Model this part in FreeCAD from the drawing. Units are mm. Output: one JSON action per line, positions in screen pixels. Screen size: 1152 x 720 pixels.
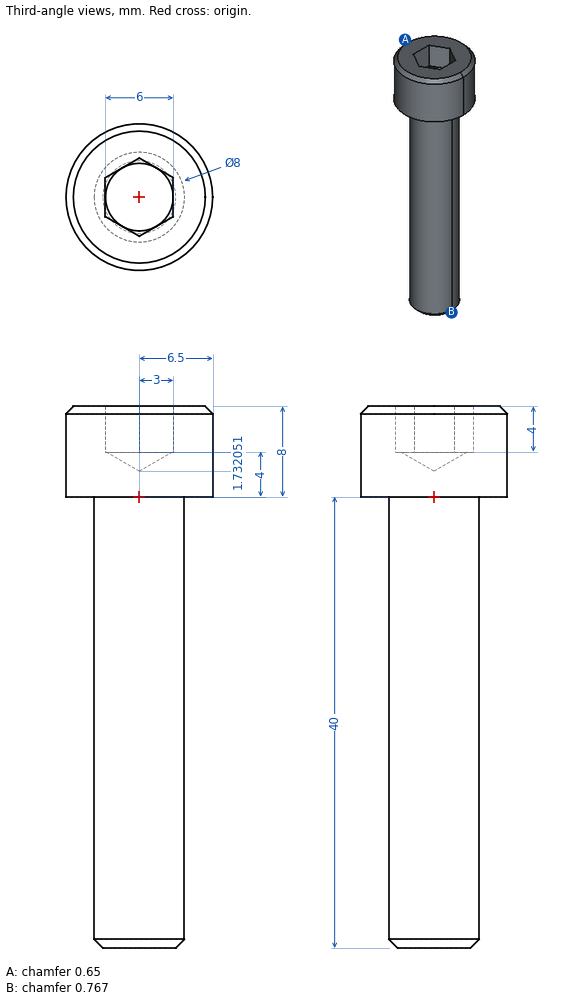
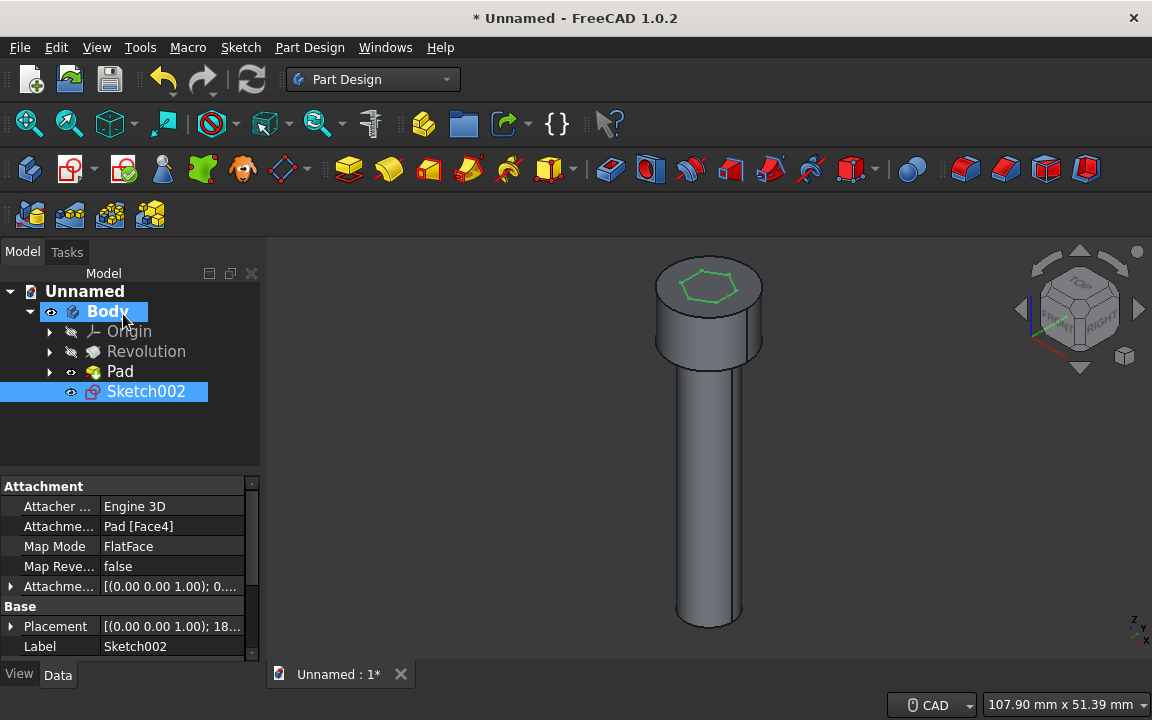
{"action": "left_click", "coordinate": [612, 170]}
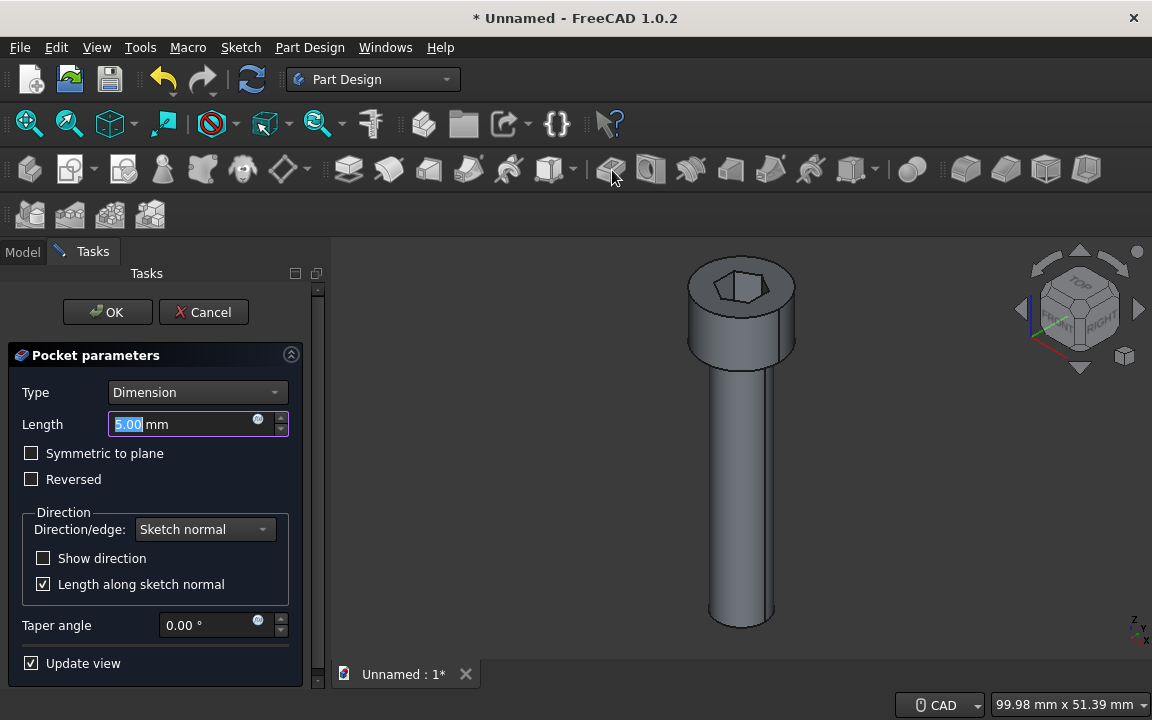
{"action": "type", "text": "4"}
{"action": "key", "text": "Tab"}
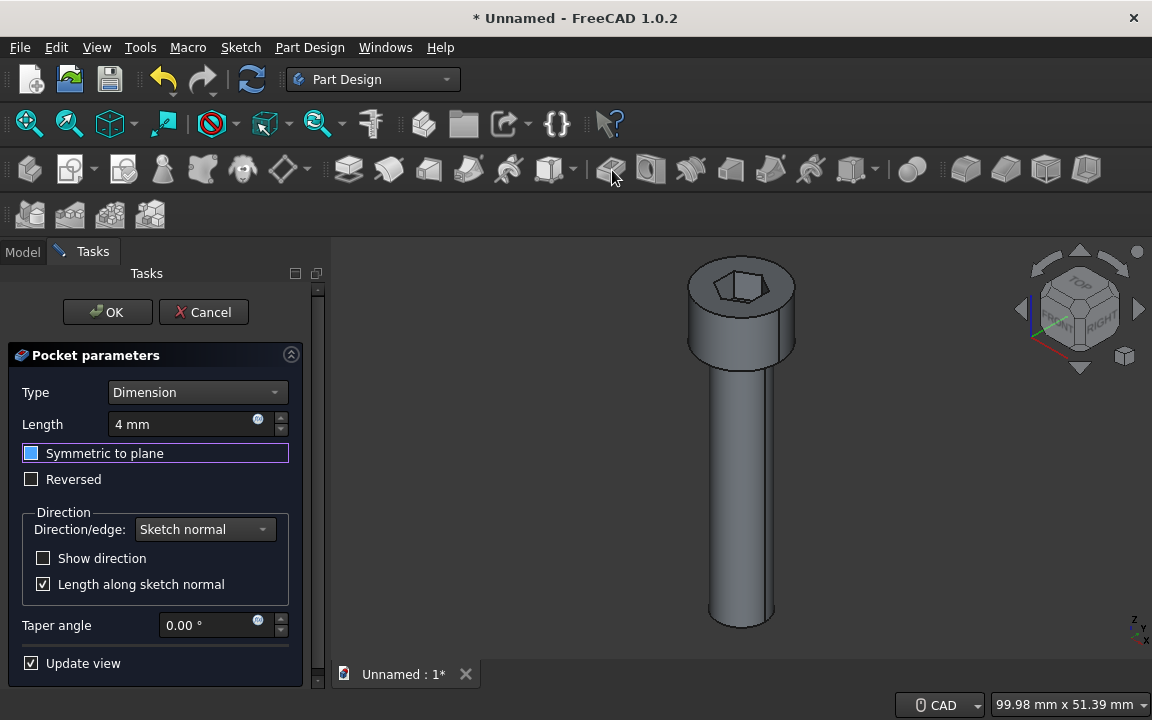
{"action": "left_click", "coordinate": [108, 312]}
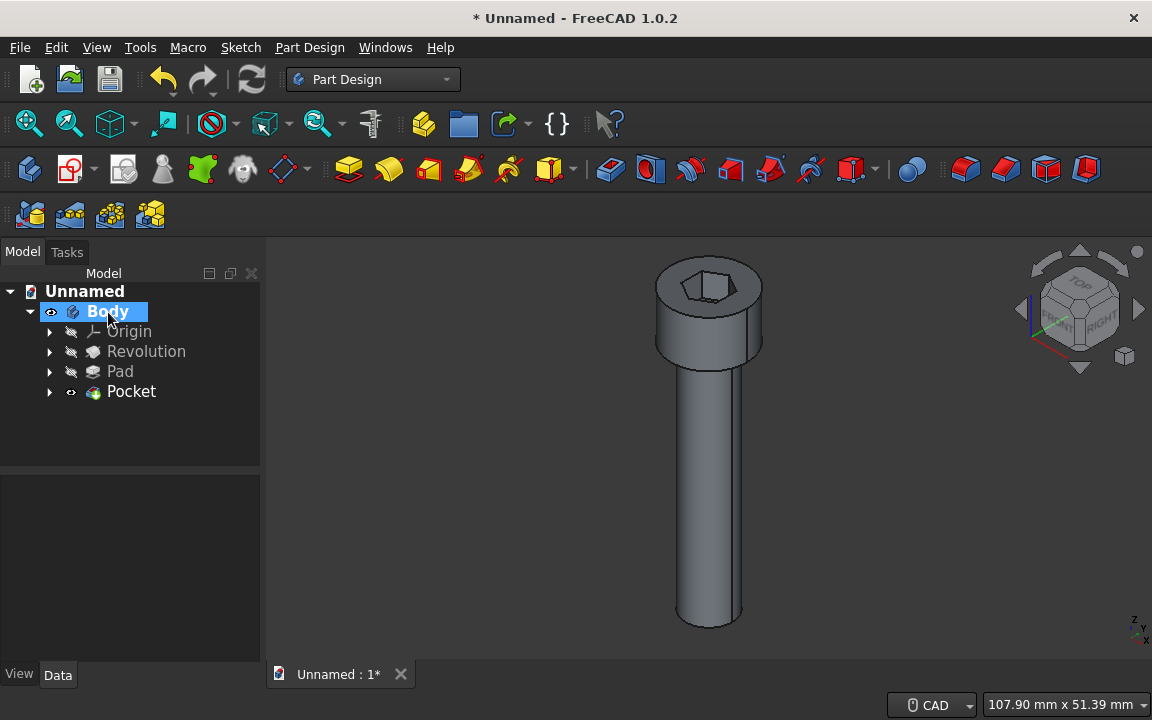
{"action": "left_click", "coordinate": [70, 170]}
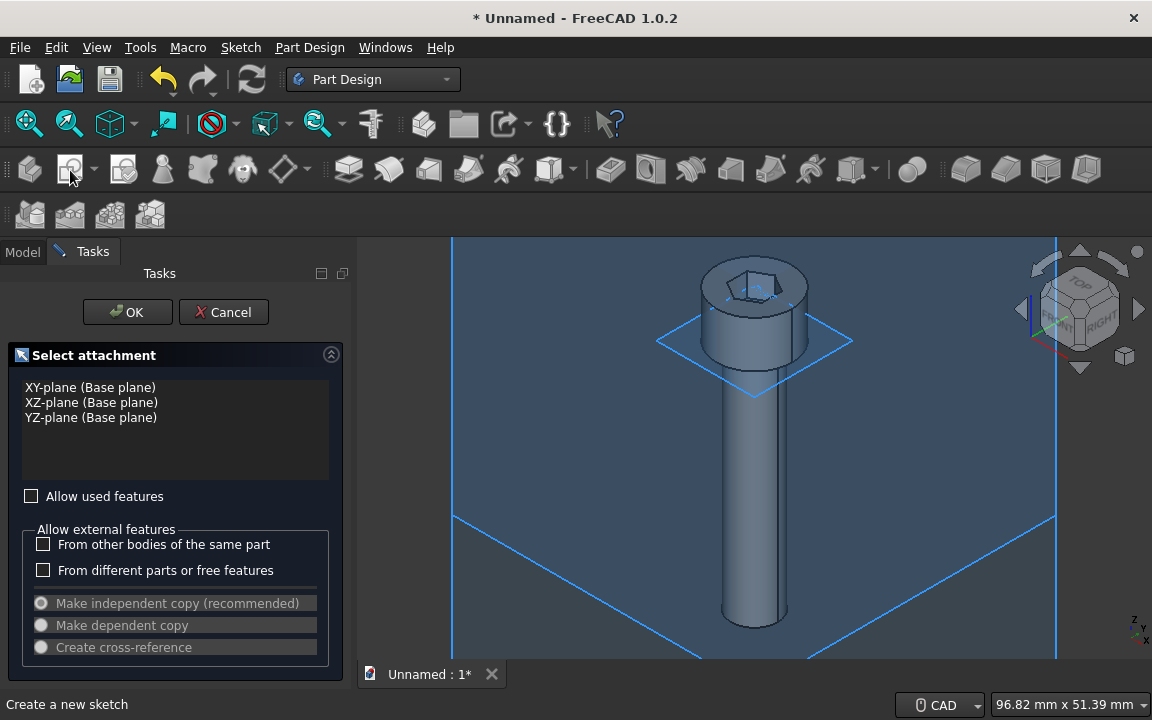
{"action": "left_click", "coordinate": [82, 402]}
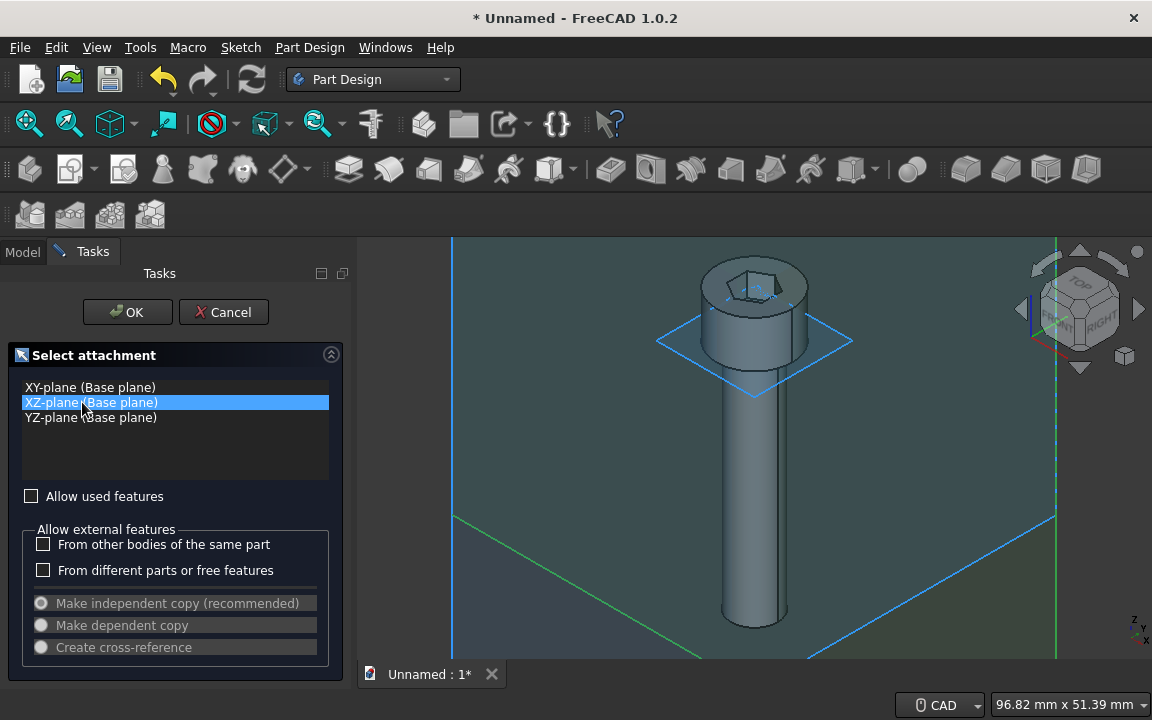
{"action": "left_click", "coordinate": [128, 312]}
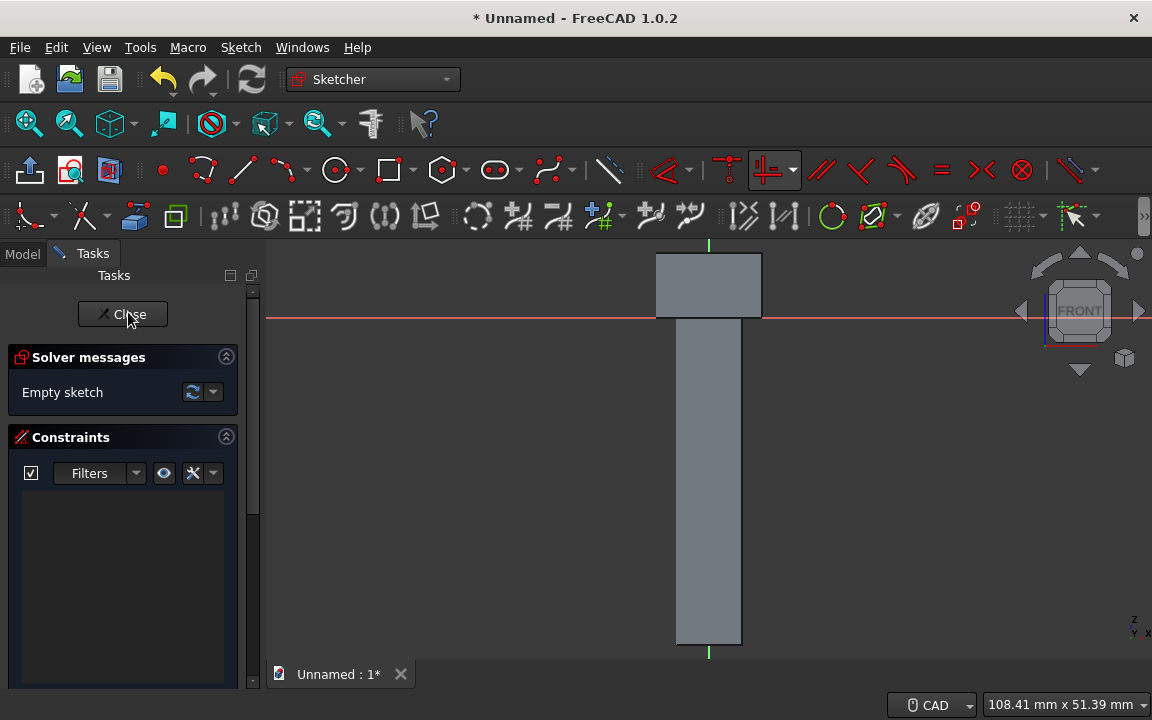
{"action": "left_click", "coordinate": [110, 170]}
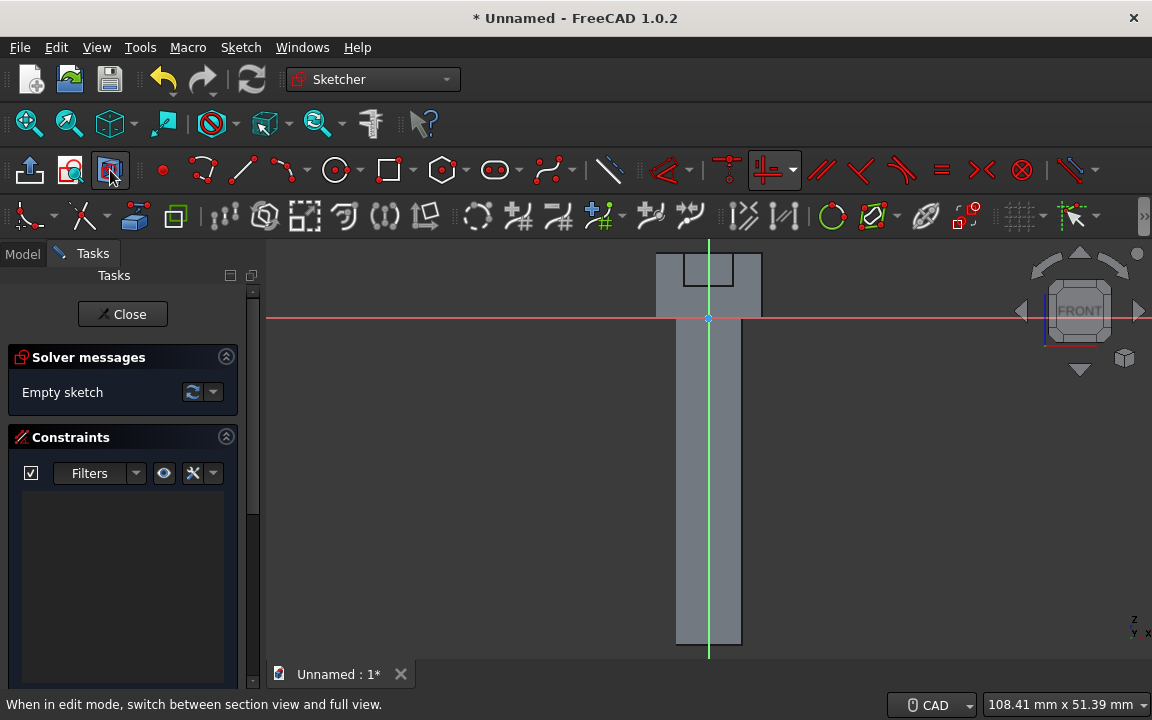
{"action": "scroll", "coordinate": [734, 279], "scroll_direction": "up", "scroll_amount": 10}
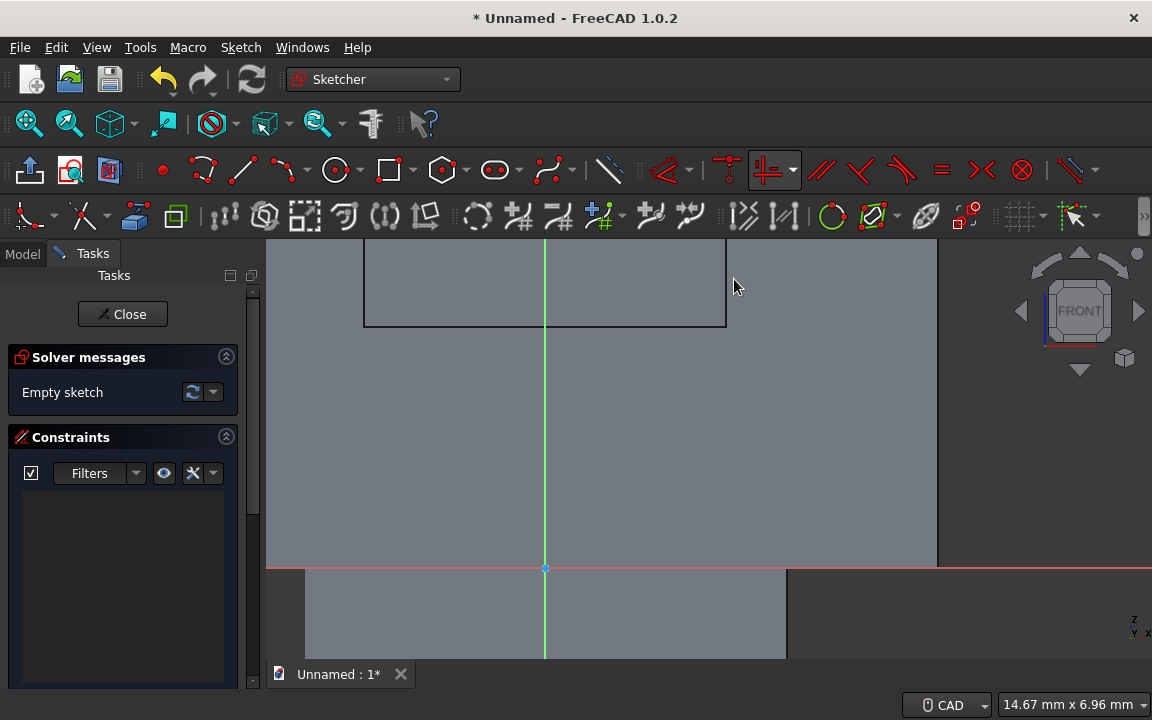
{"action": "left_click", "coordinate": [204, 170]}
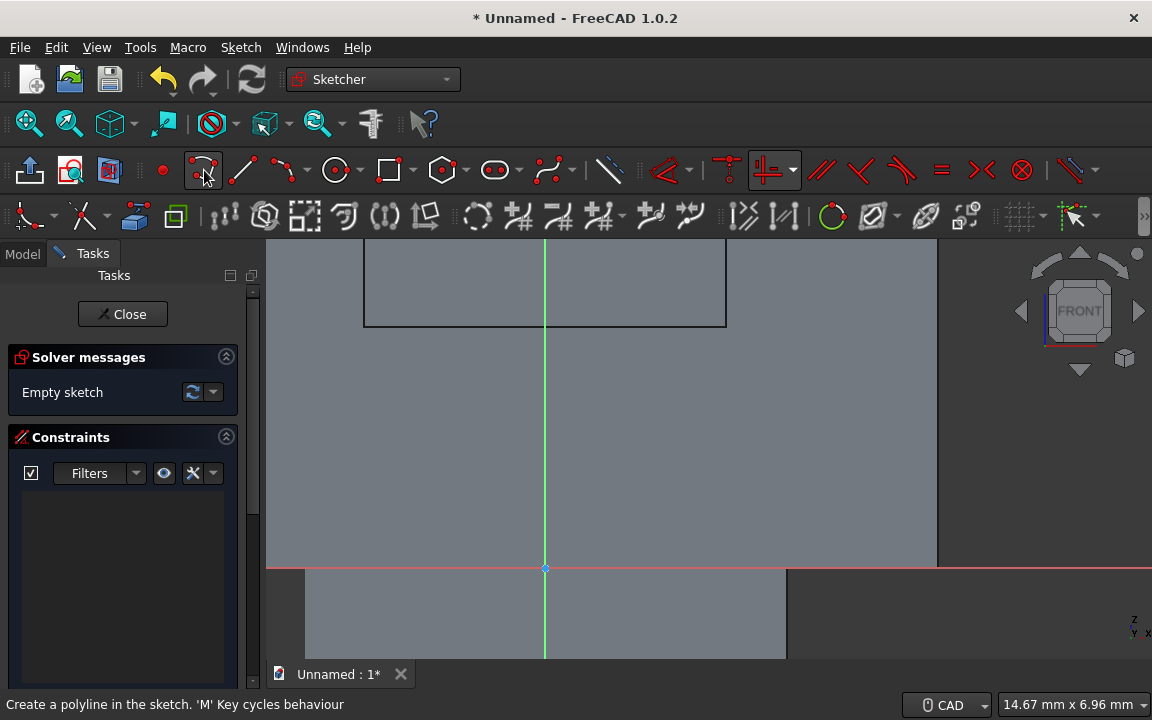
{"action": "left_click", "coordinate": [545, 431]}
{"action": "left_click", "coordinate": [726, 327]}
{"action": "left_click", "coordinate": [554, 327]}
{"action": "left_click", "coordinate": [545, 432]}
{"action": "key", "text": "Escape"}
{"action": "key", "text": "Escape"}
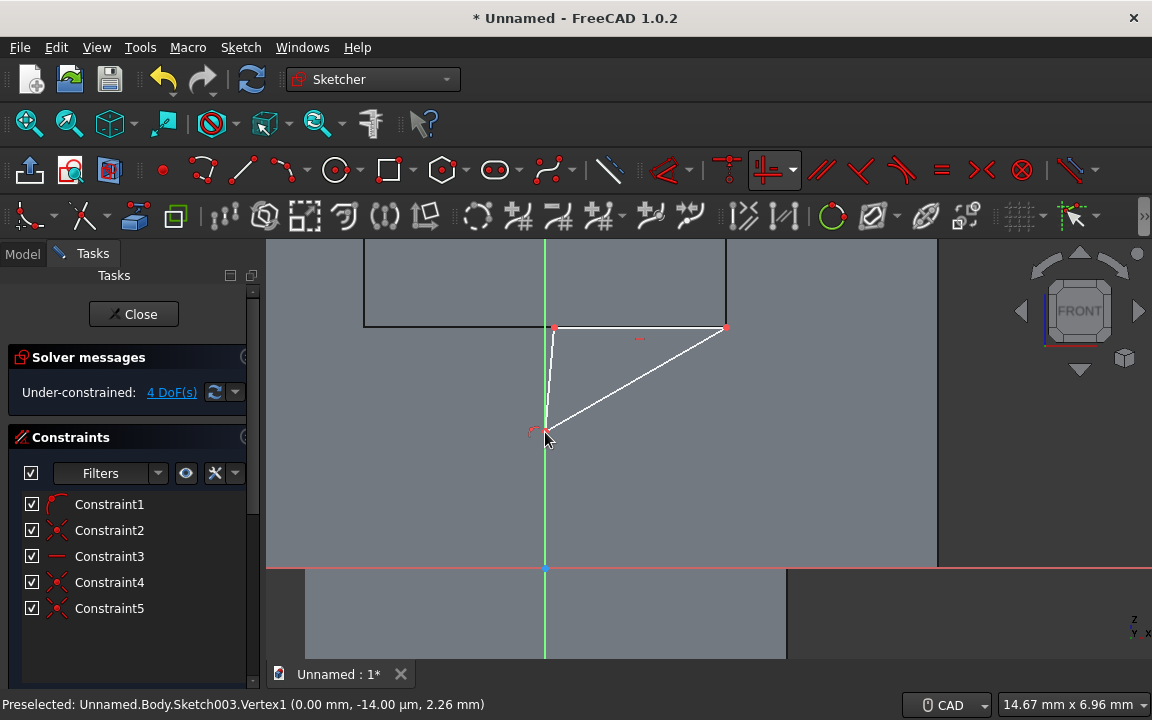
{"action": "left_click", "coordinate": [548, 401]}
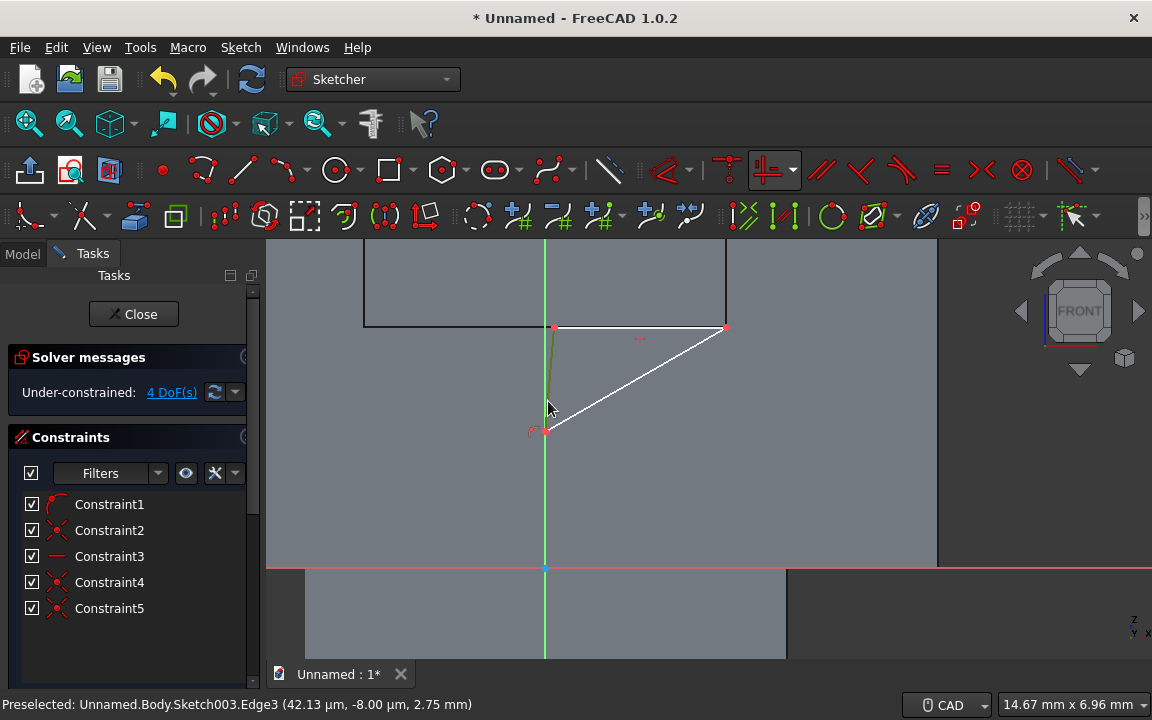
{"action": "left_click", "coordinate": [796, 170]}